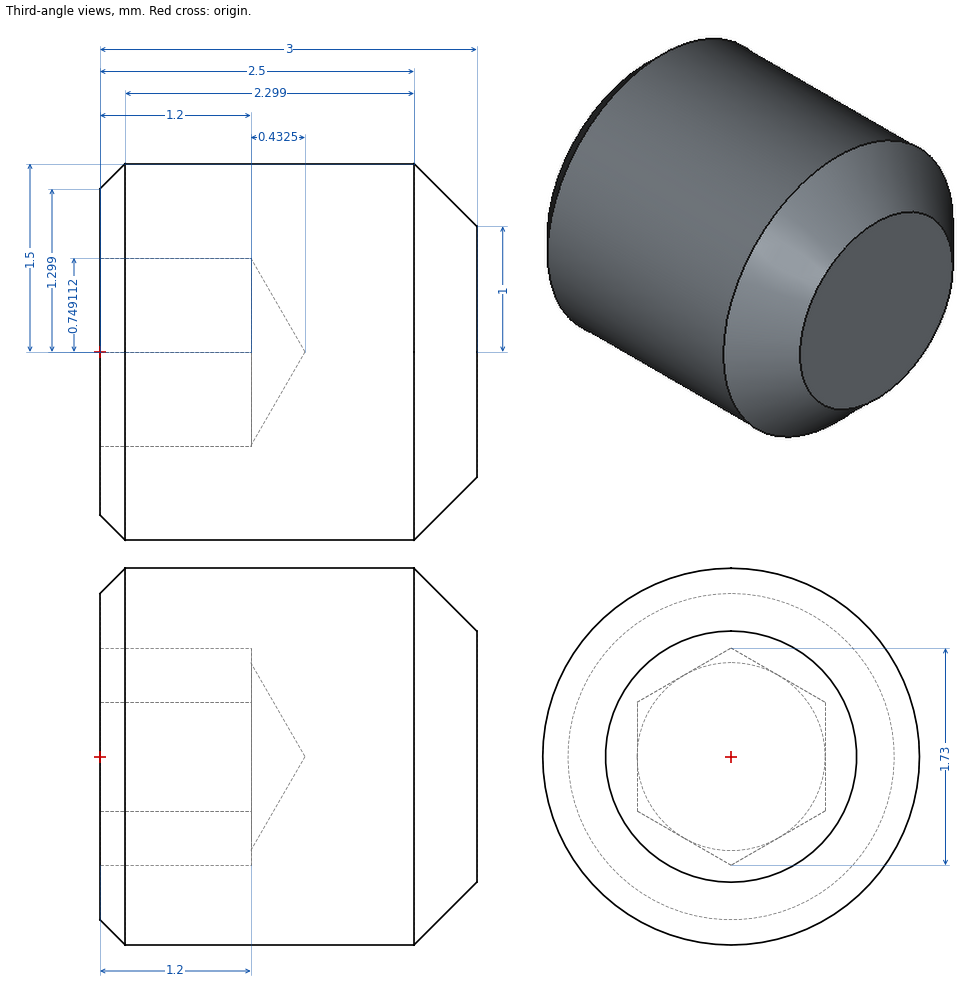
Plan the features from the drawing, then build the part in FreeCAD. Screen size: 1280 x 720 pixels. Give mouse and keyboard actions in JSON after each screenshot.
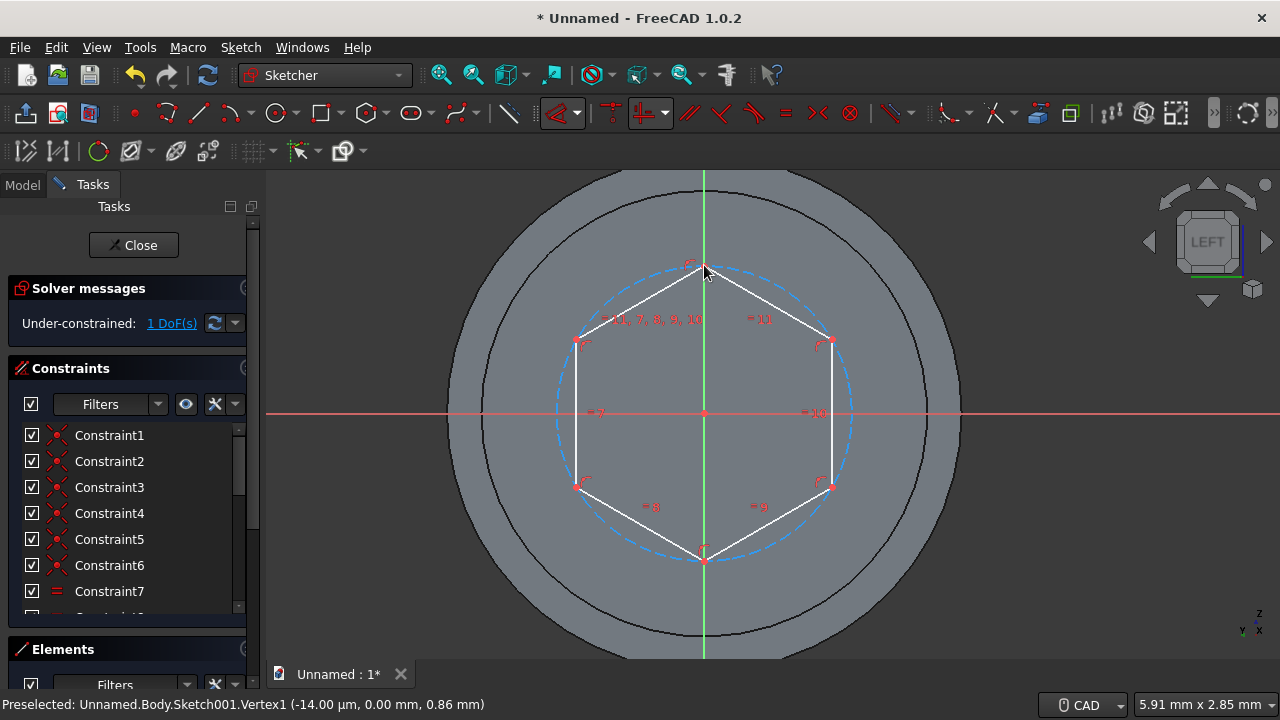
{"action": "left_click", "coordinate": [704, 561]}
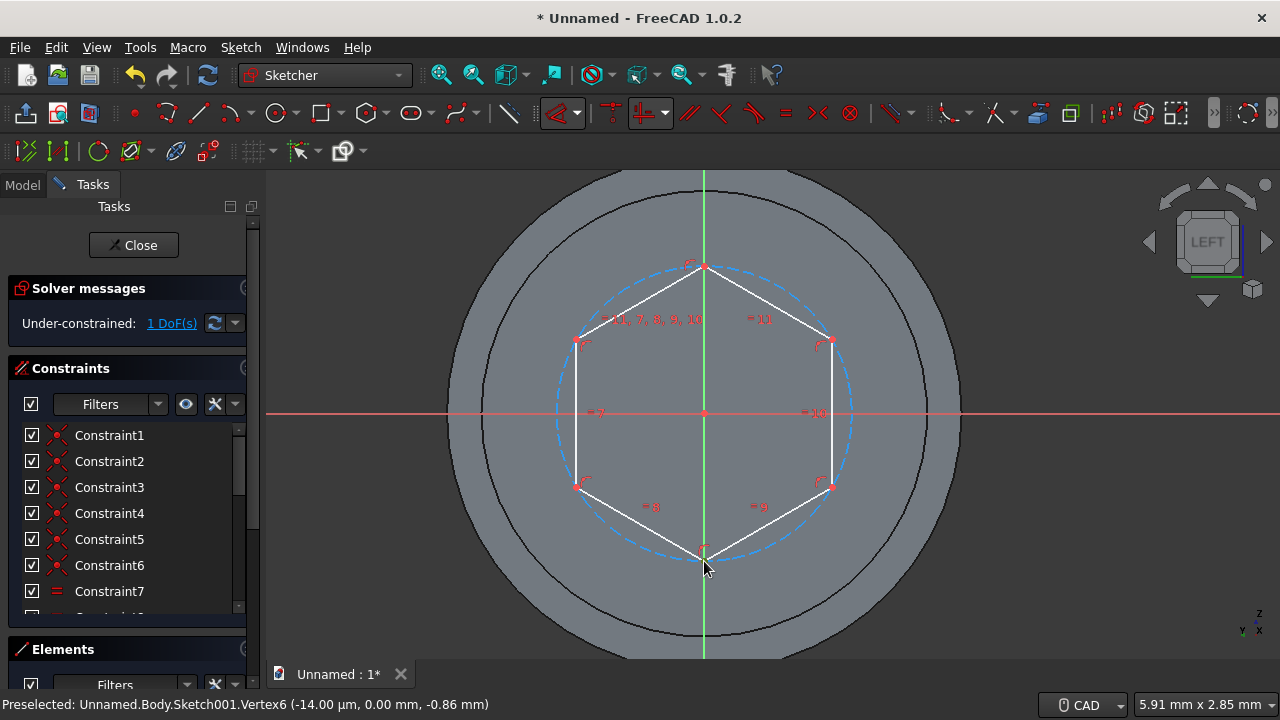
{"action": "left_click", "coordinate": [704, 266]}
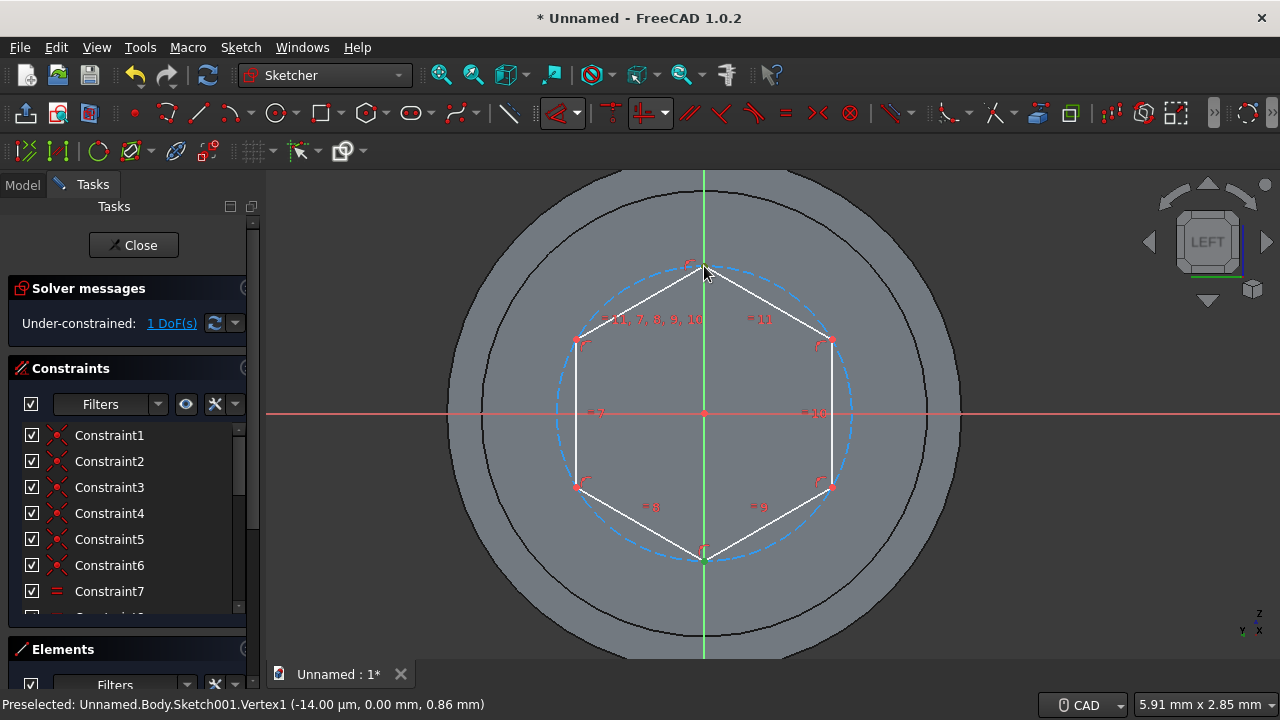
{"action": "key", "text": "i"}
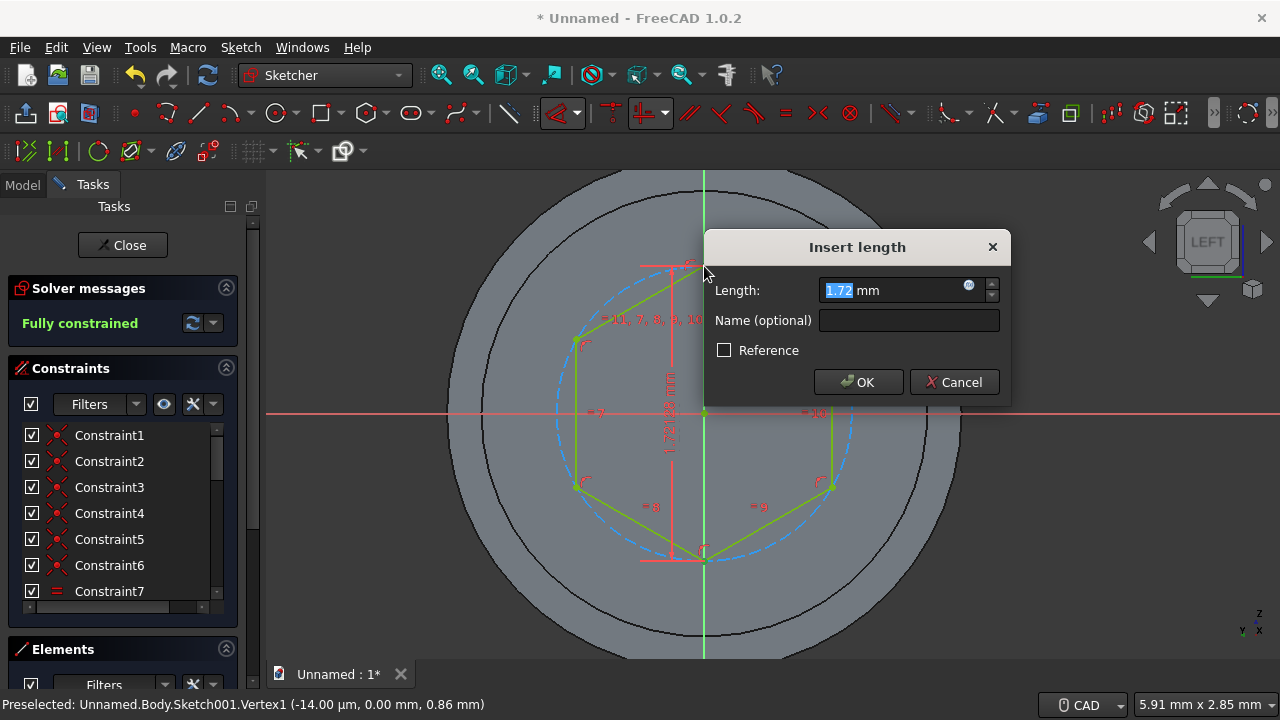
{"action": "type", "text": "1.73"}
{"action": "key", "text": "Return"}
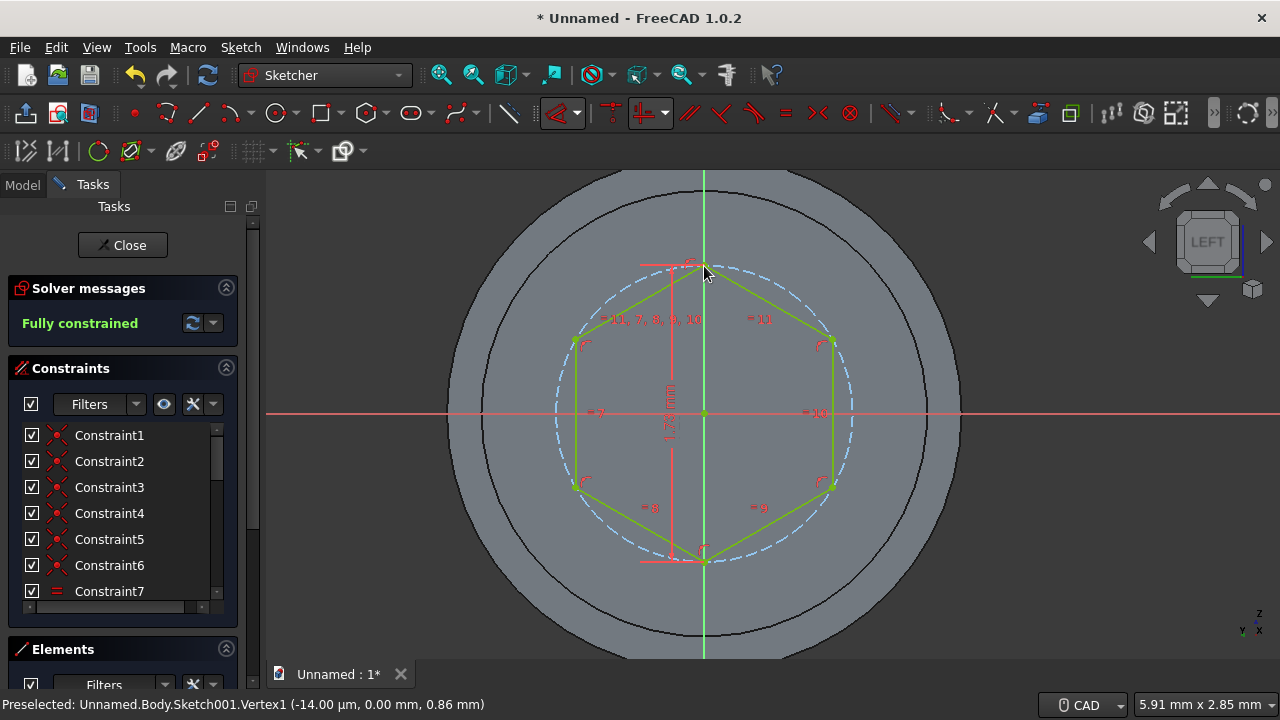
{"action": "left_click", "coordinate": [123, 245]}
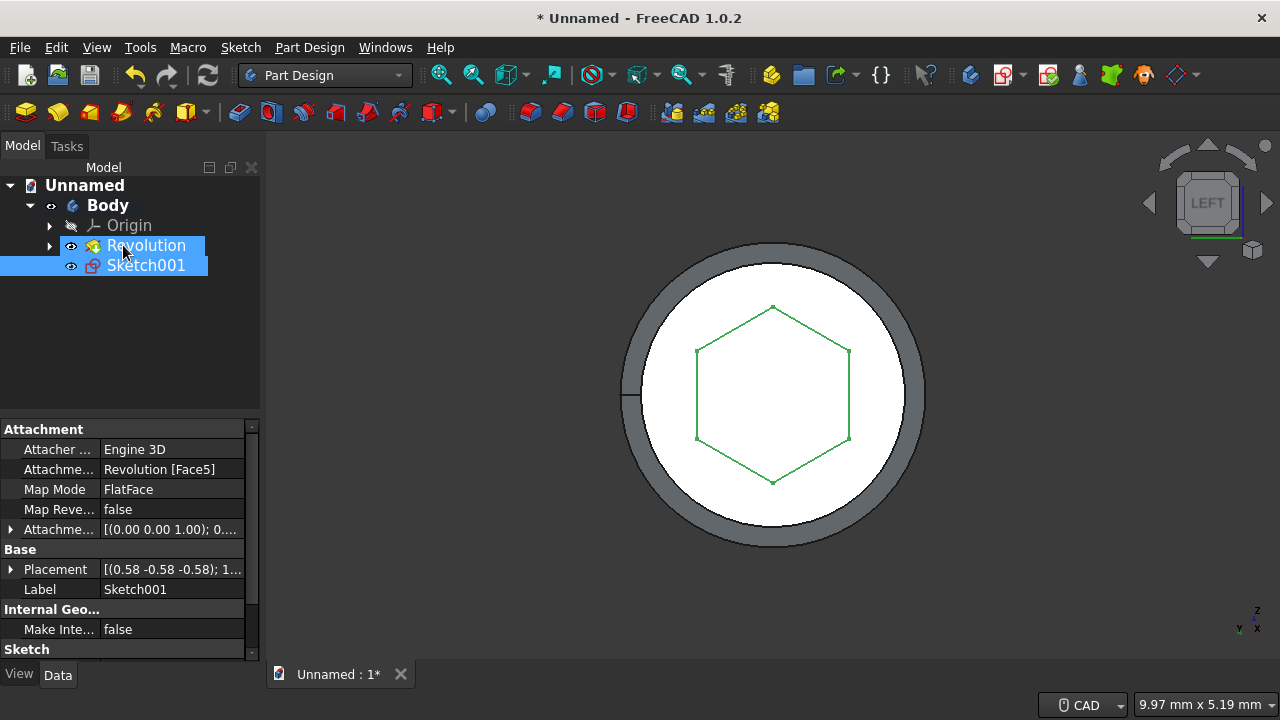
{"action": "left_click", "coordinate": [240, 112]}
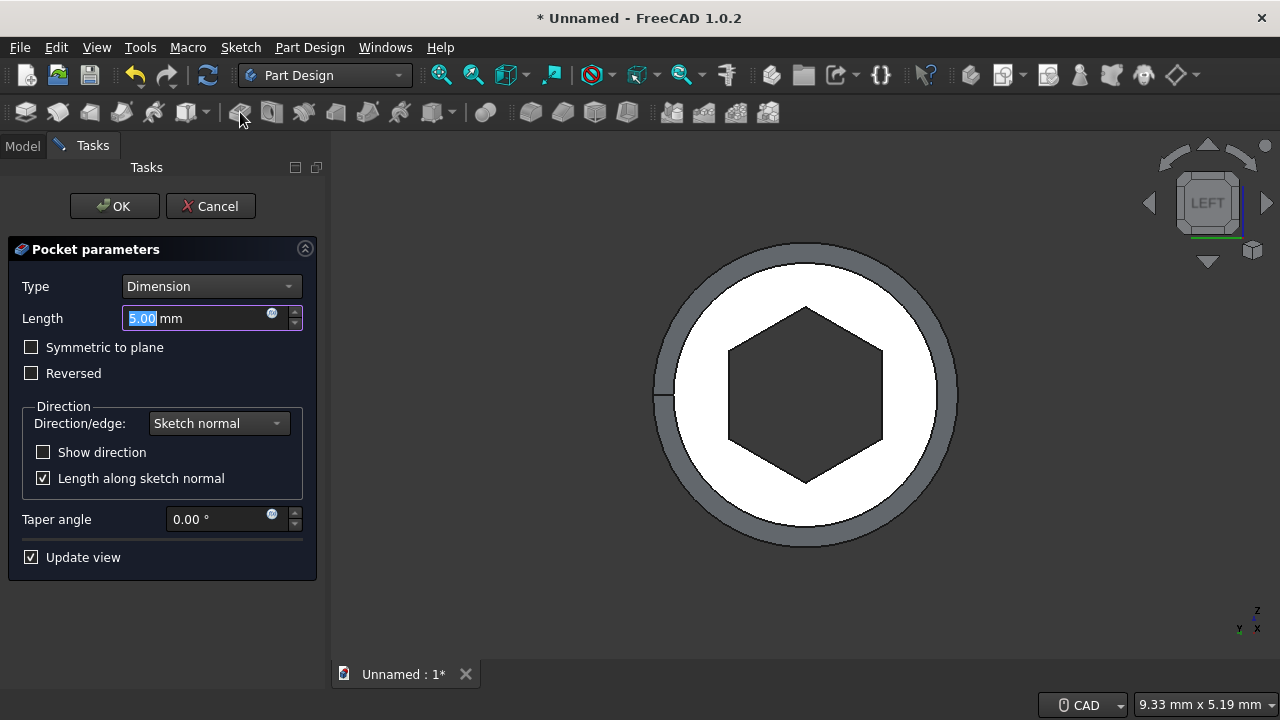
{"action": "type", "text": "1.2"}
{"action": "key", "text": "Tab"}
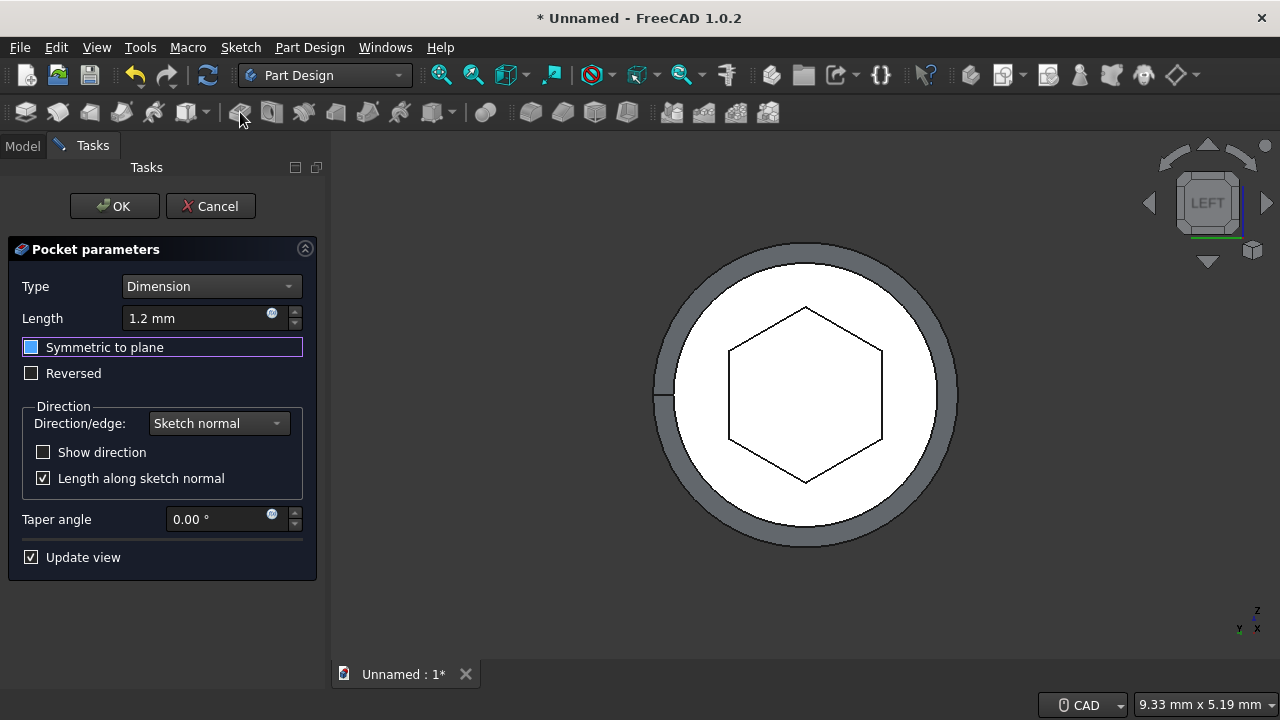
{"action": "left_click", "coordinate": [115, 206]}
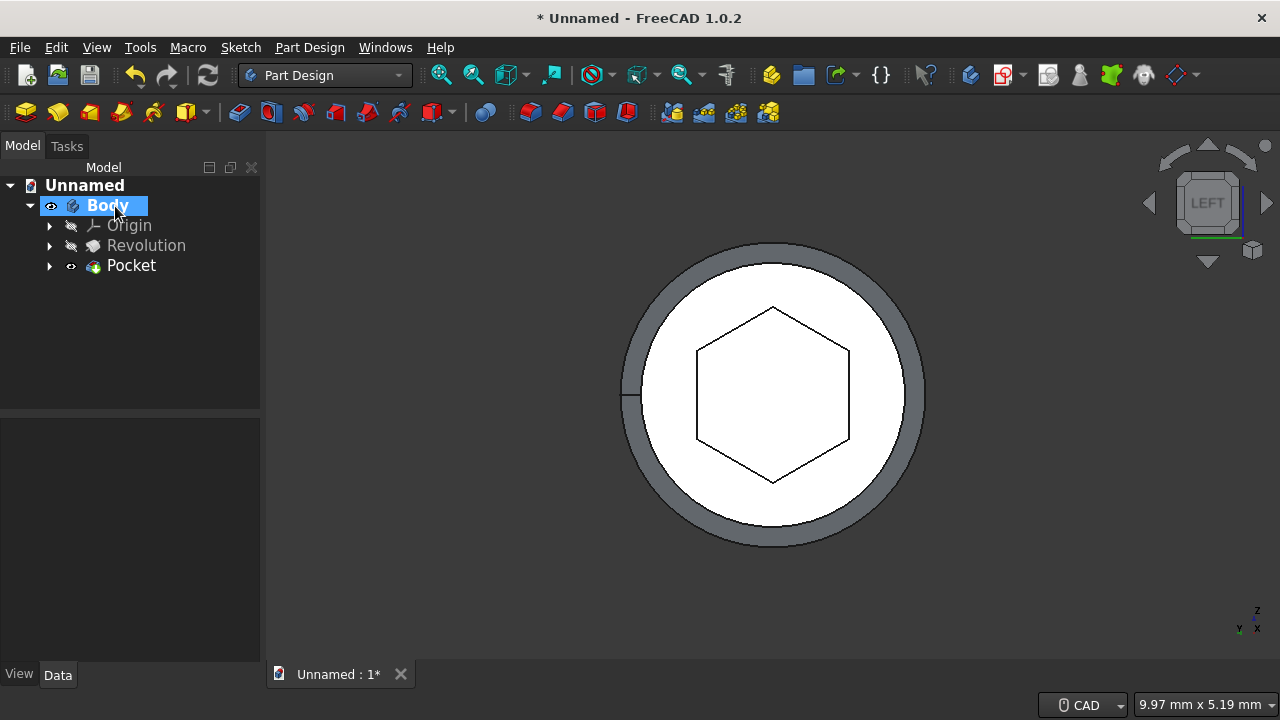
{"action": "left_click", "coordinate": [1004, 76]}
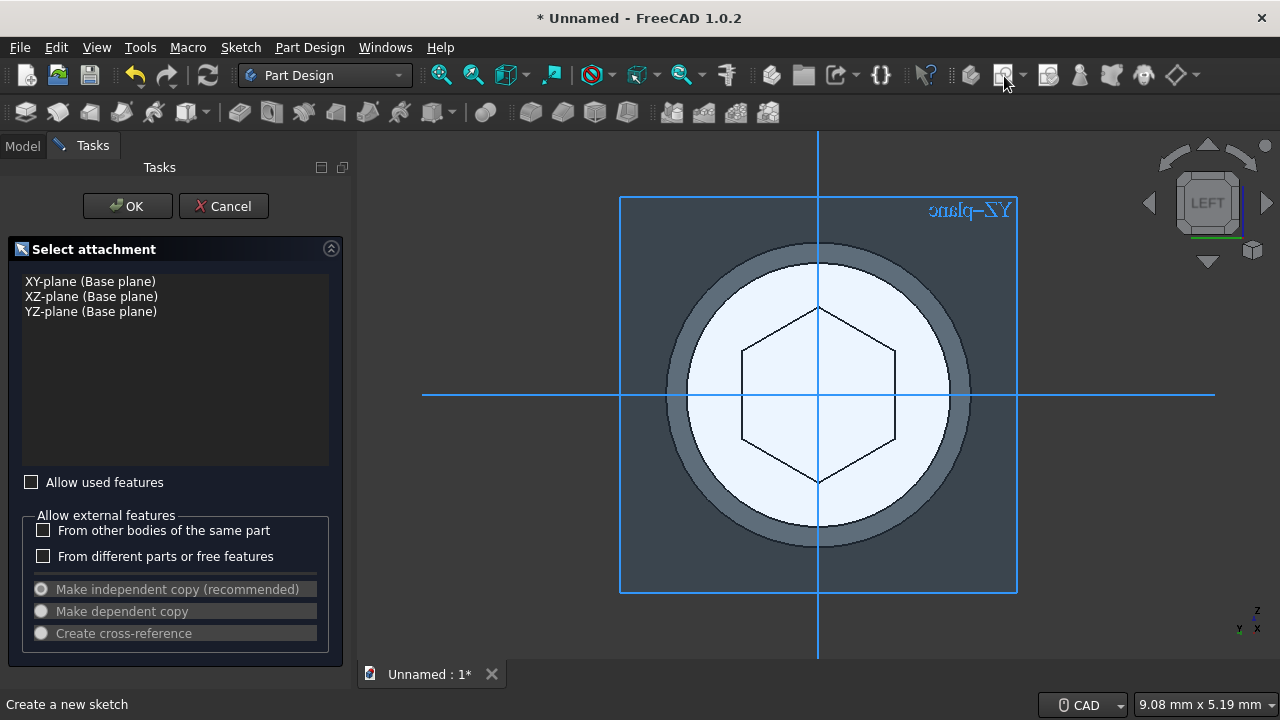
{"action": "left_click", "coordinate": [82, 282]}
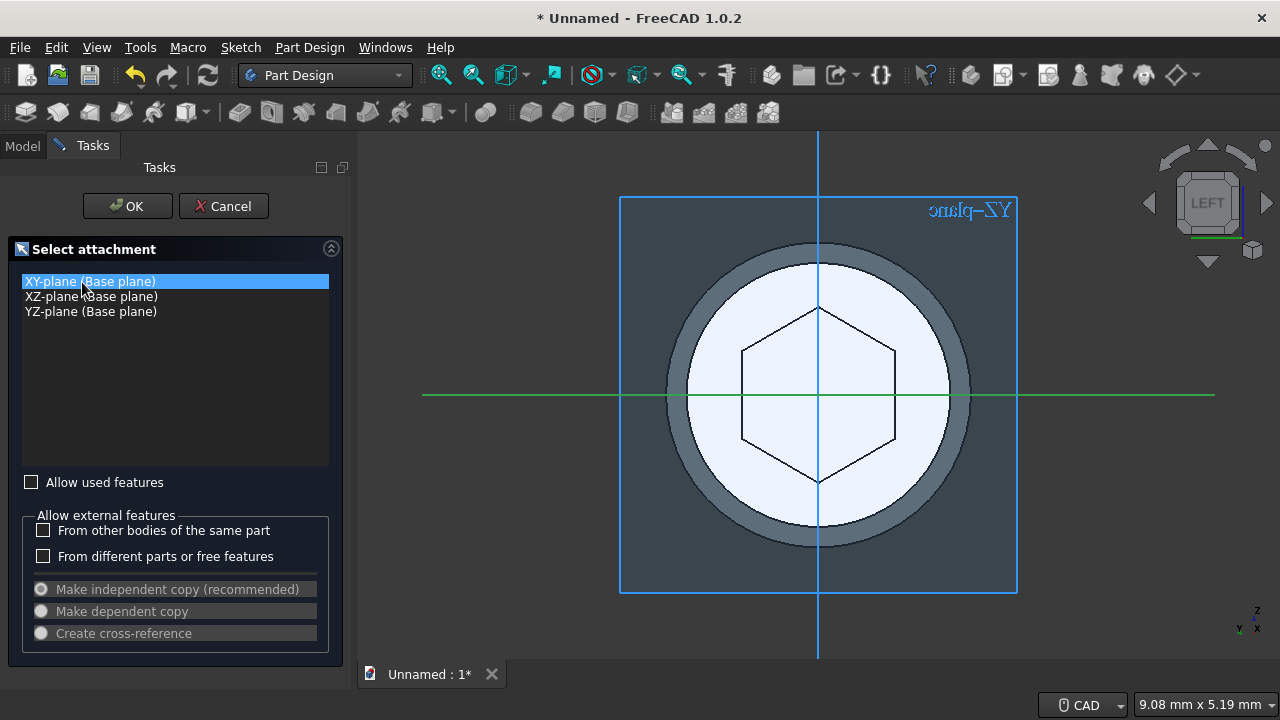
{"action": "left_click", "coordinate": [128, 206]}